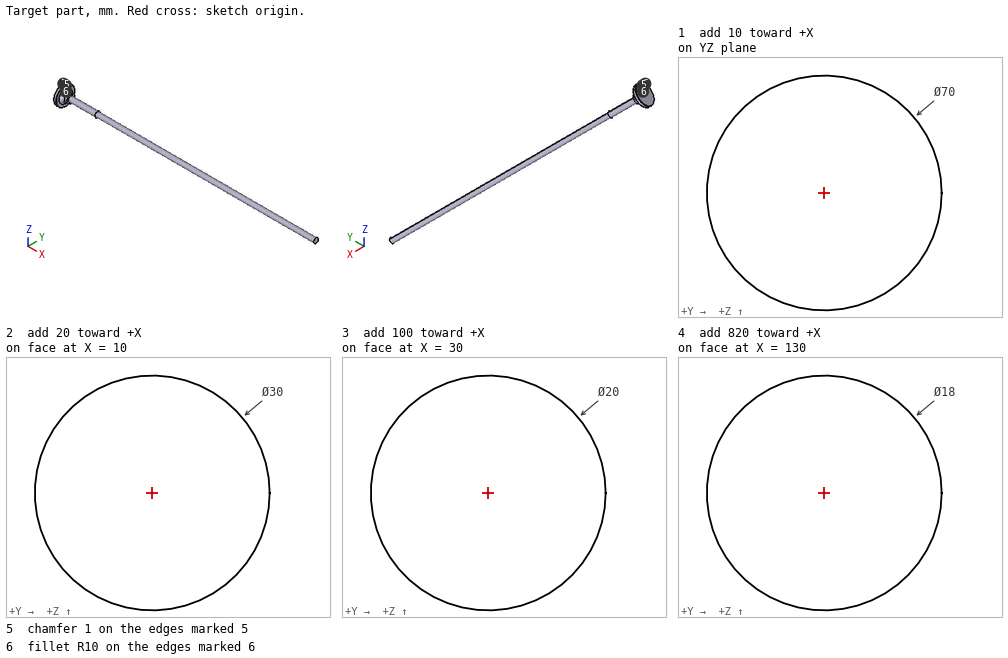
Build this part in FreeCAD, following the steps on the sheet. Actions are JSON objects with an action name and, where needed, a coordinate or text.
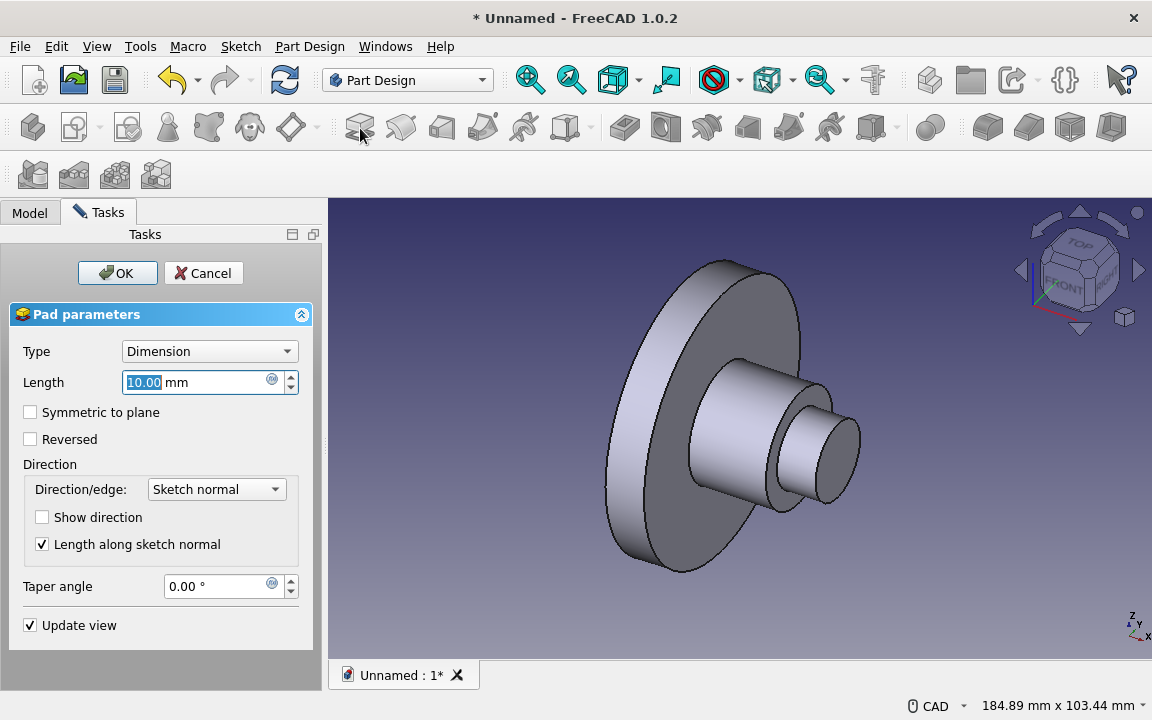
{"action": "type", "text": "100"}
{"action": "key", "text": "Tab"}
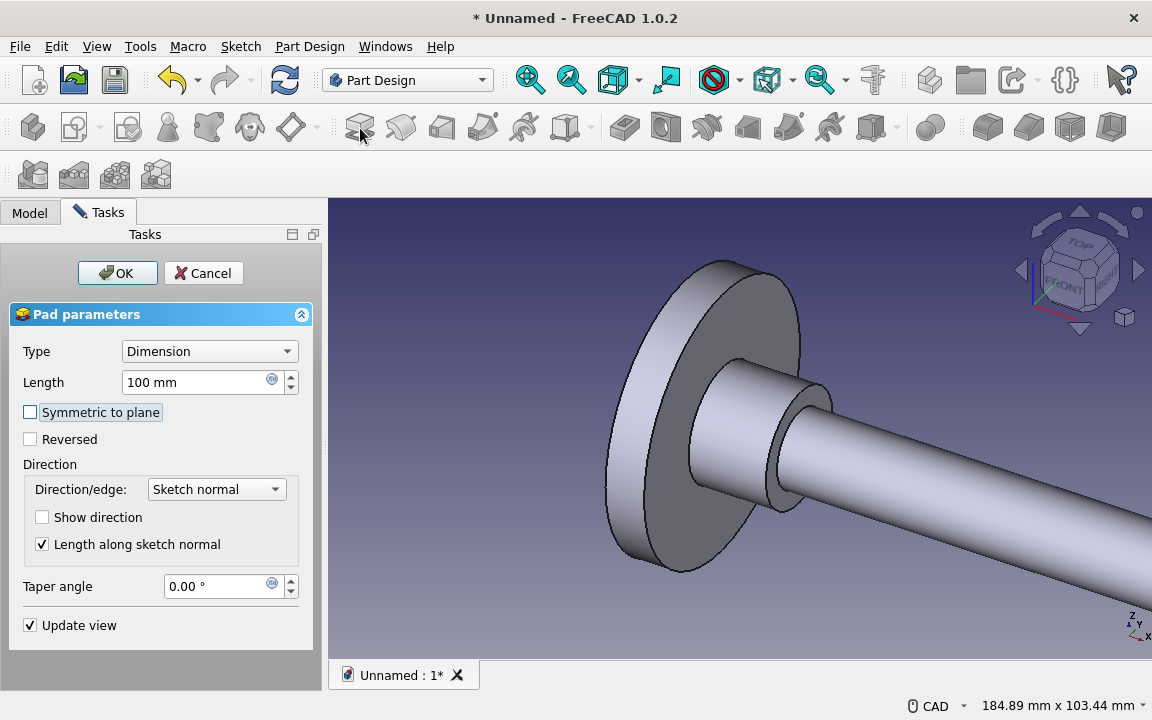
{"action": "left_click", "coordinate": [118, 273]}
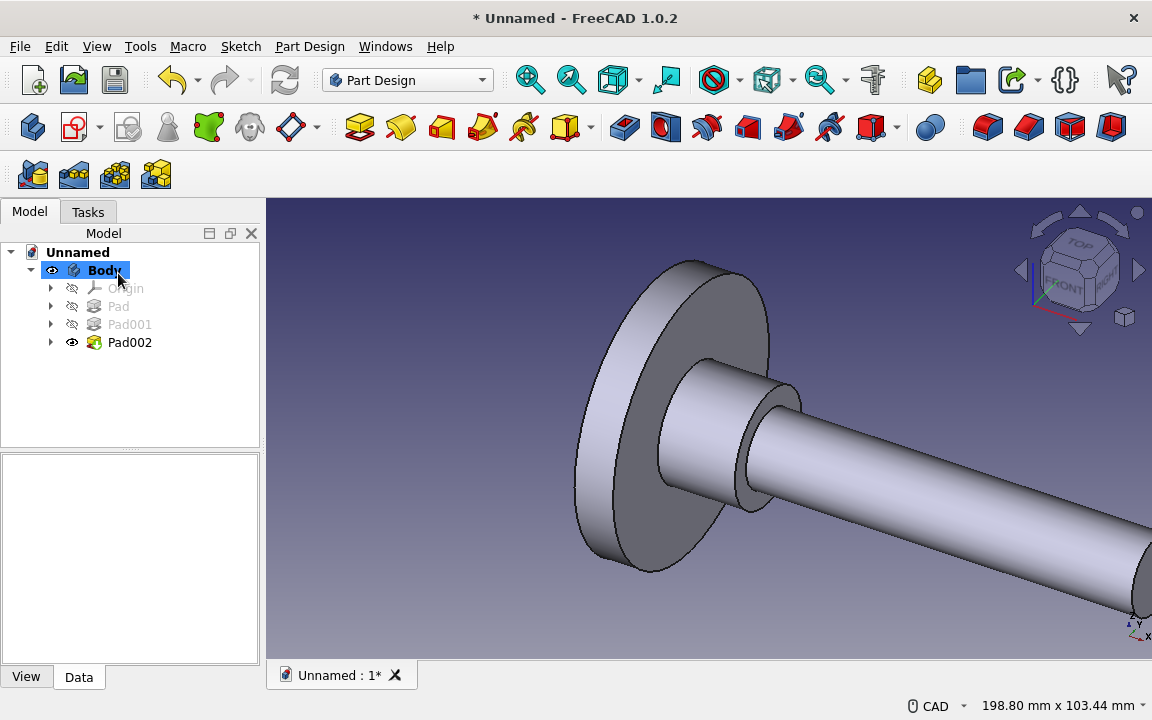
{"action": "key", "text": "v f"}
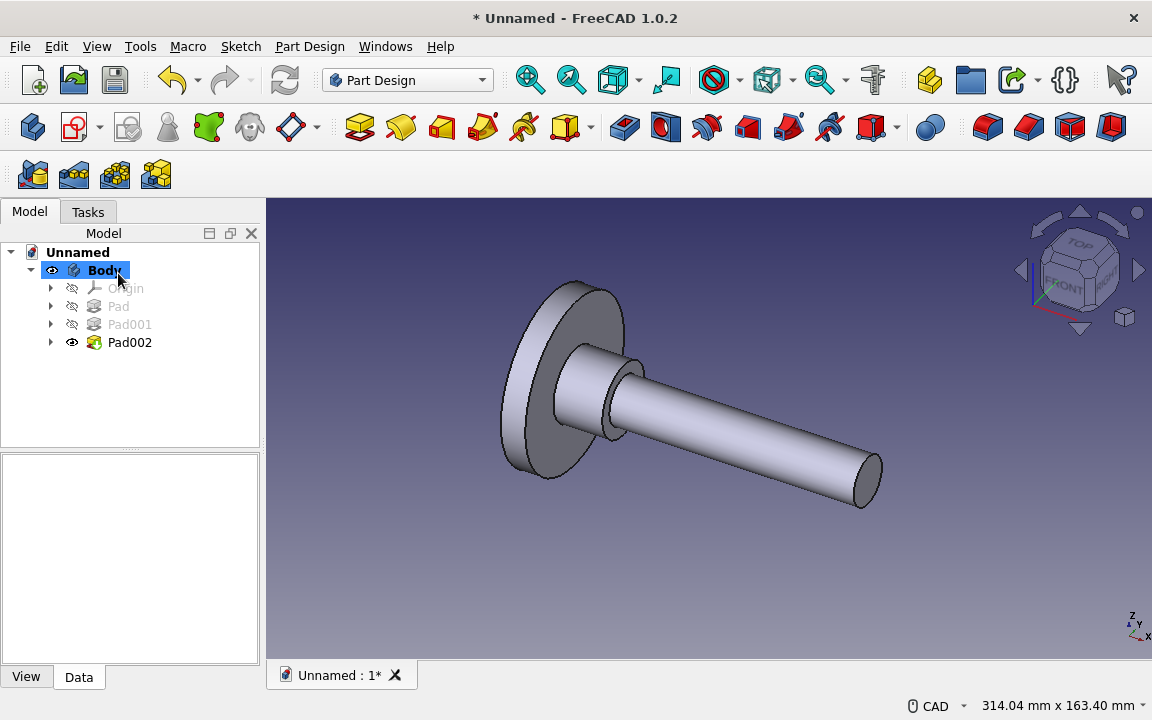
{"action": "left_click", "coordinate": [868, 480]}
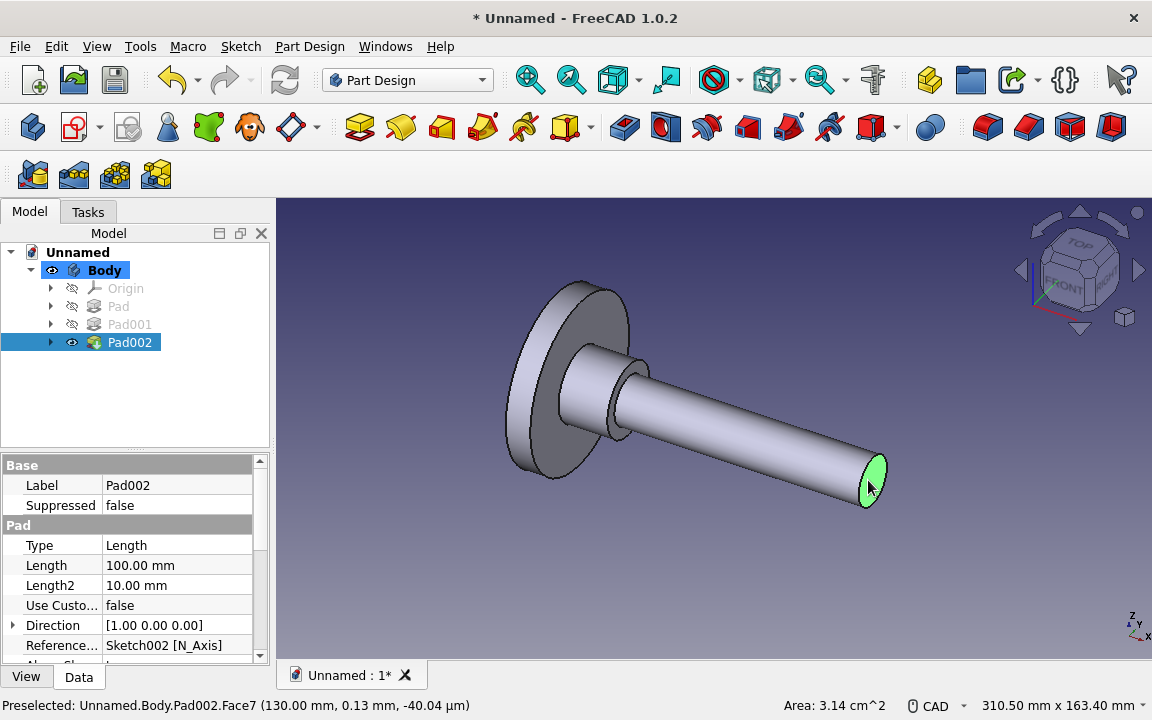
{"action": "left_click", "coordinate": [74, 128]}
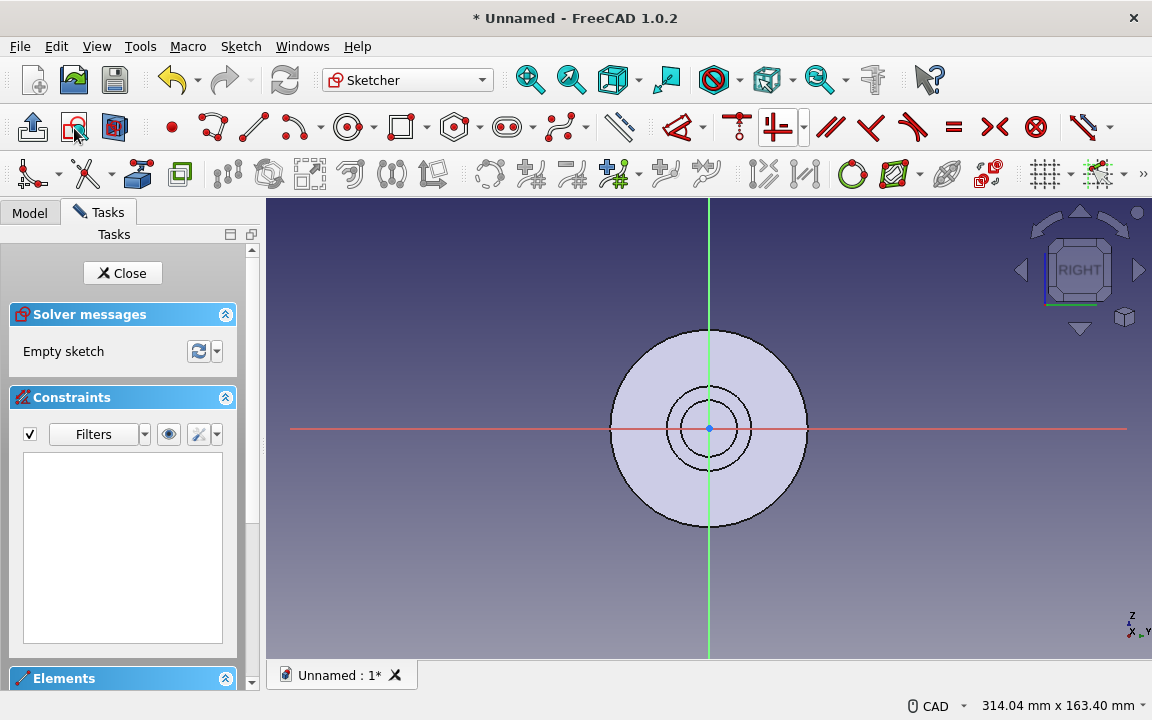
{"action": "scroll", "coordinate": [723, 428], "scroll_direction": "up", "scroll_amount": 9}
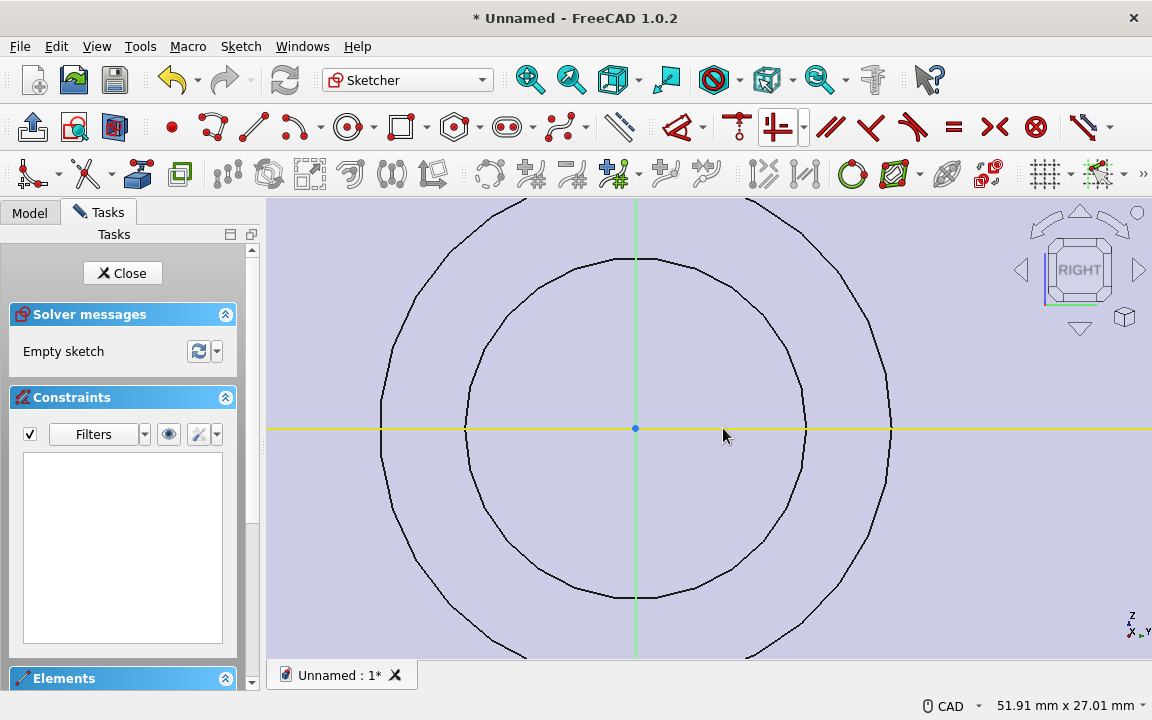
{"action": "left_click", "coordinate": [348, 128]}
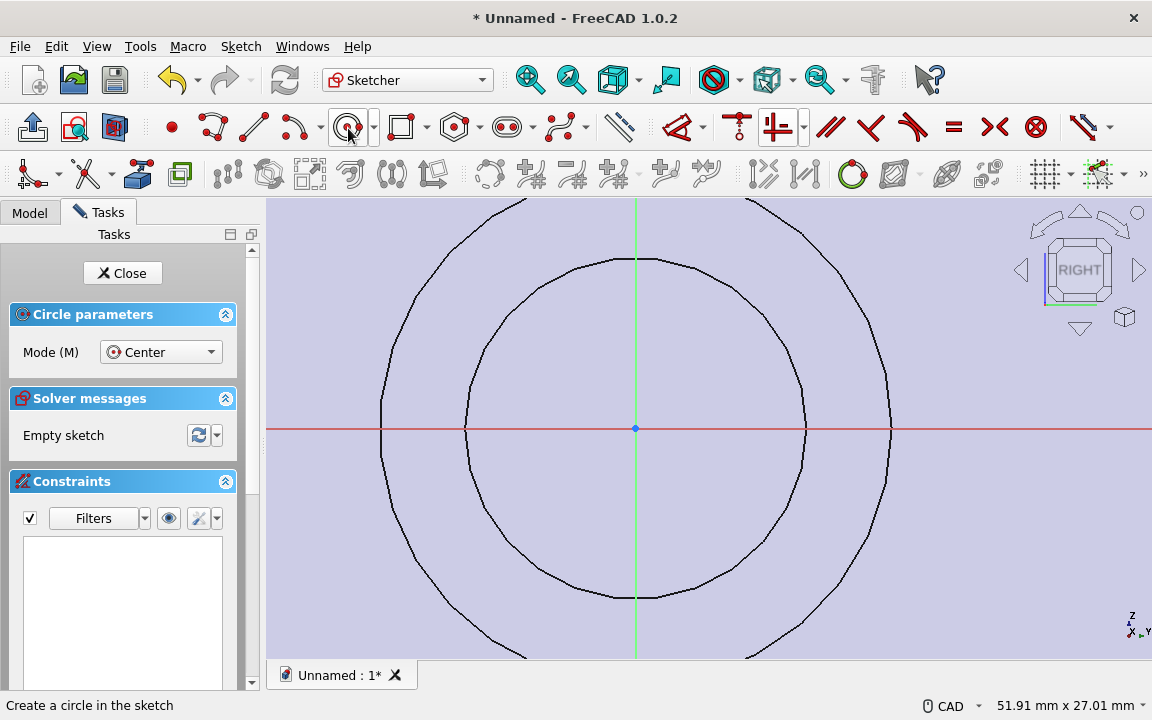
{"action": "left_click", "coordinate": [636, 428]}
{"action": "left_click", "coordinate": [744, 320]}
{"action": "key", "text": "Escape"}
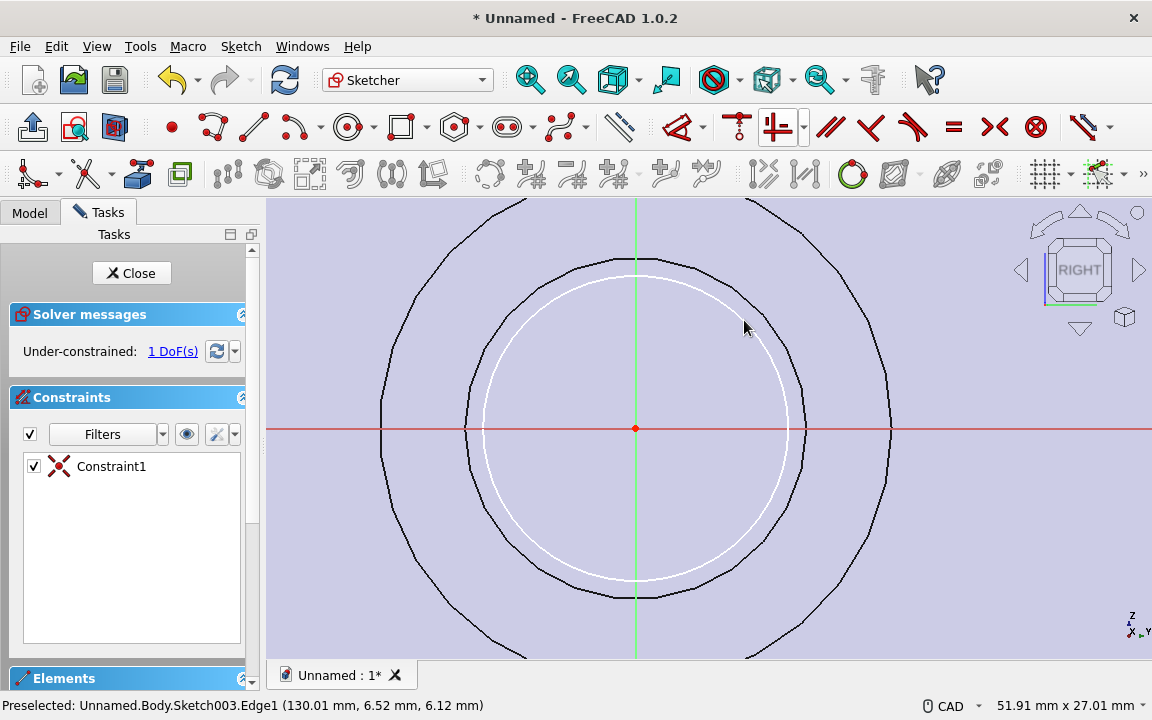
{"action": "key", "text": "d"}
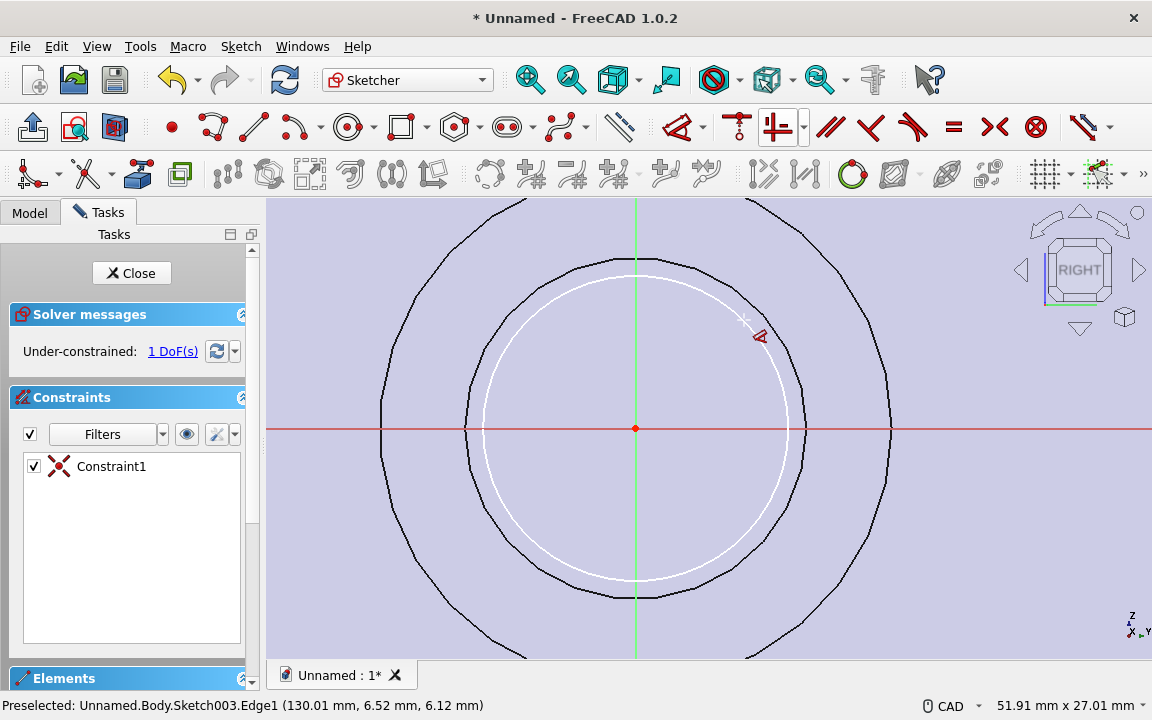
{"action": "left_click", "coordinate": [743, 320]}
{"action": "left_click", "coordinate": [766, 297]}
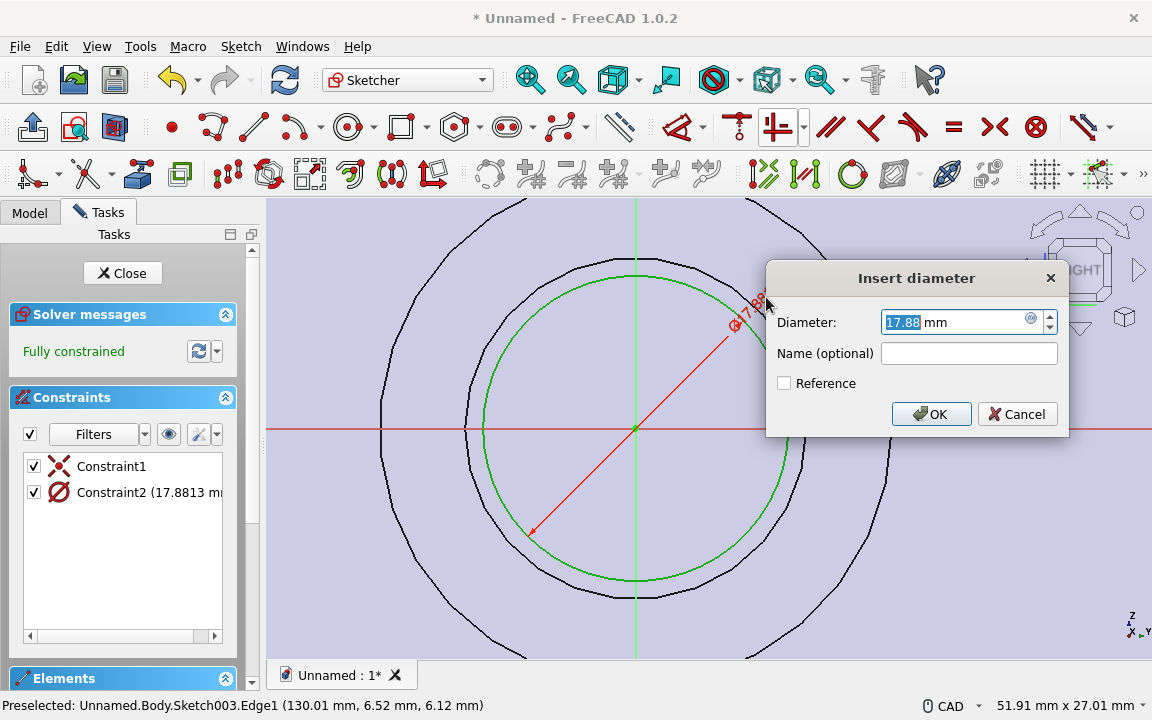
{"action": "type", "text": "18"}
{"action": "key", "text": "Return"}
{"action": "key", "text": "Escape"}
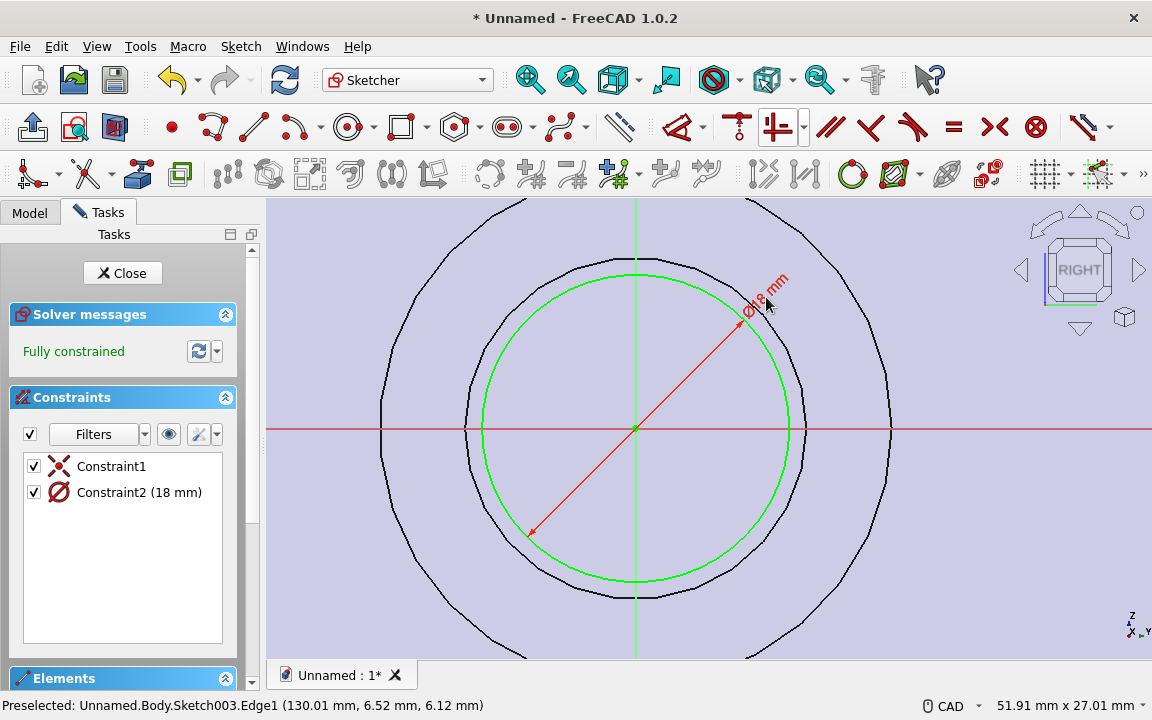
{"action": "left_click", "coordinate": [123, 273]}